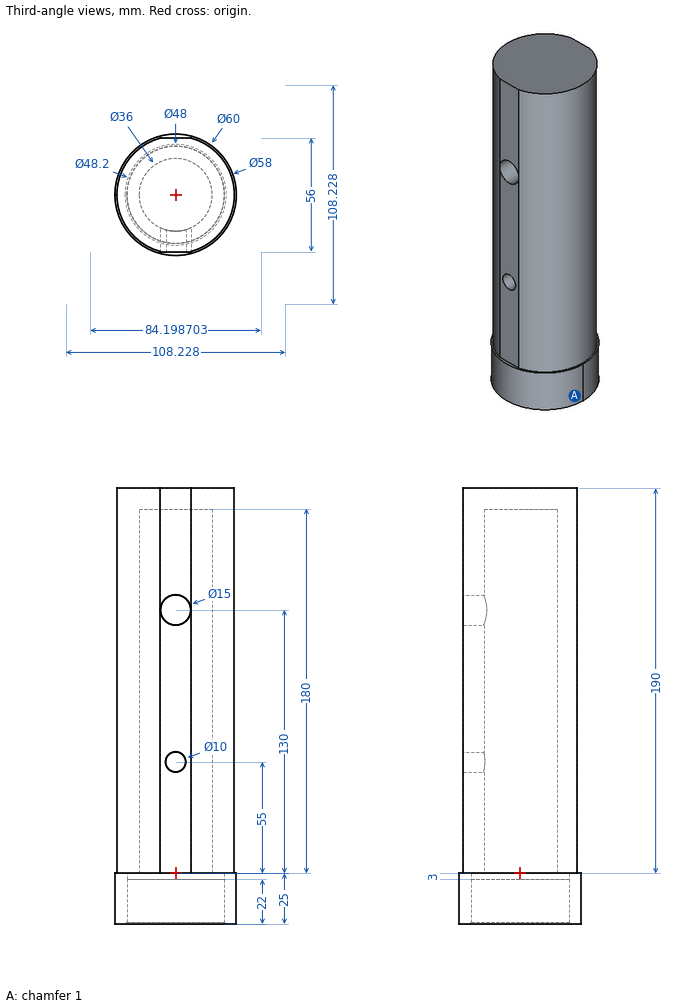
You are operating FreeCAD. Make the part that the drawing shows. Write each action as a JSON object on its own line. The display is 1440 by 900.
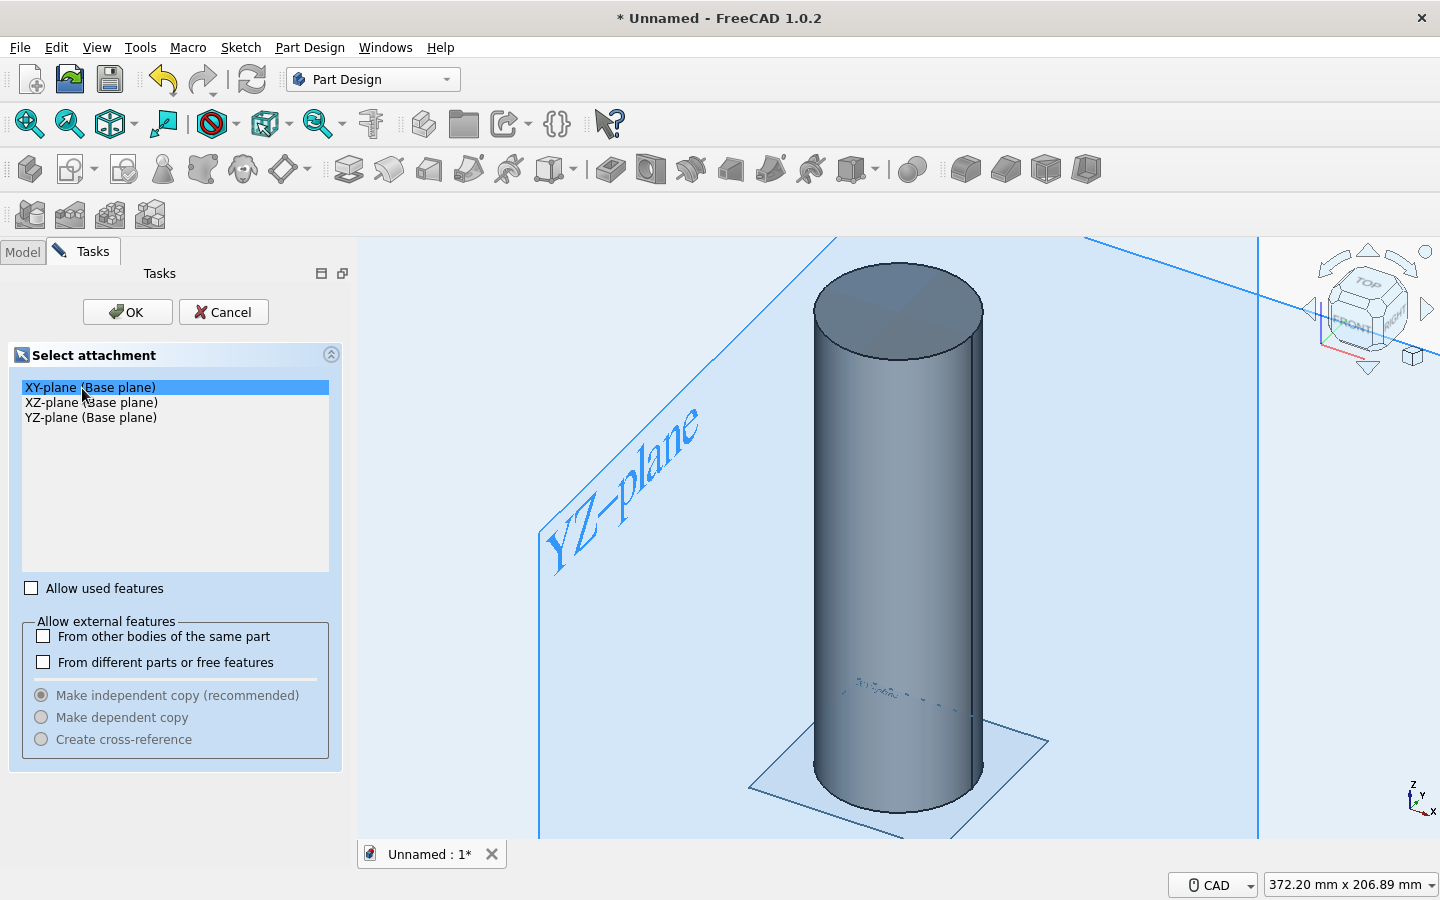
{"action": "left_click", "coordinate": [128, 312]}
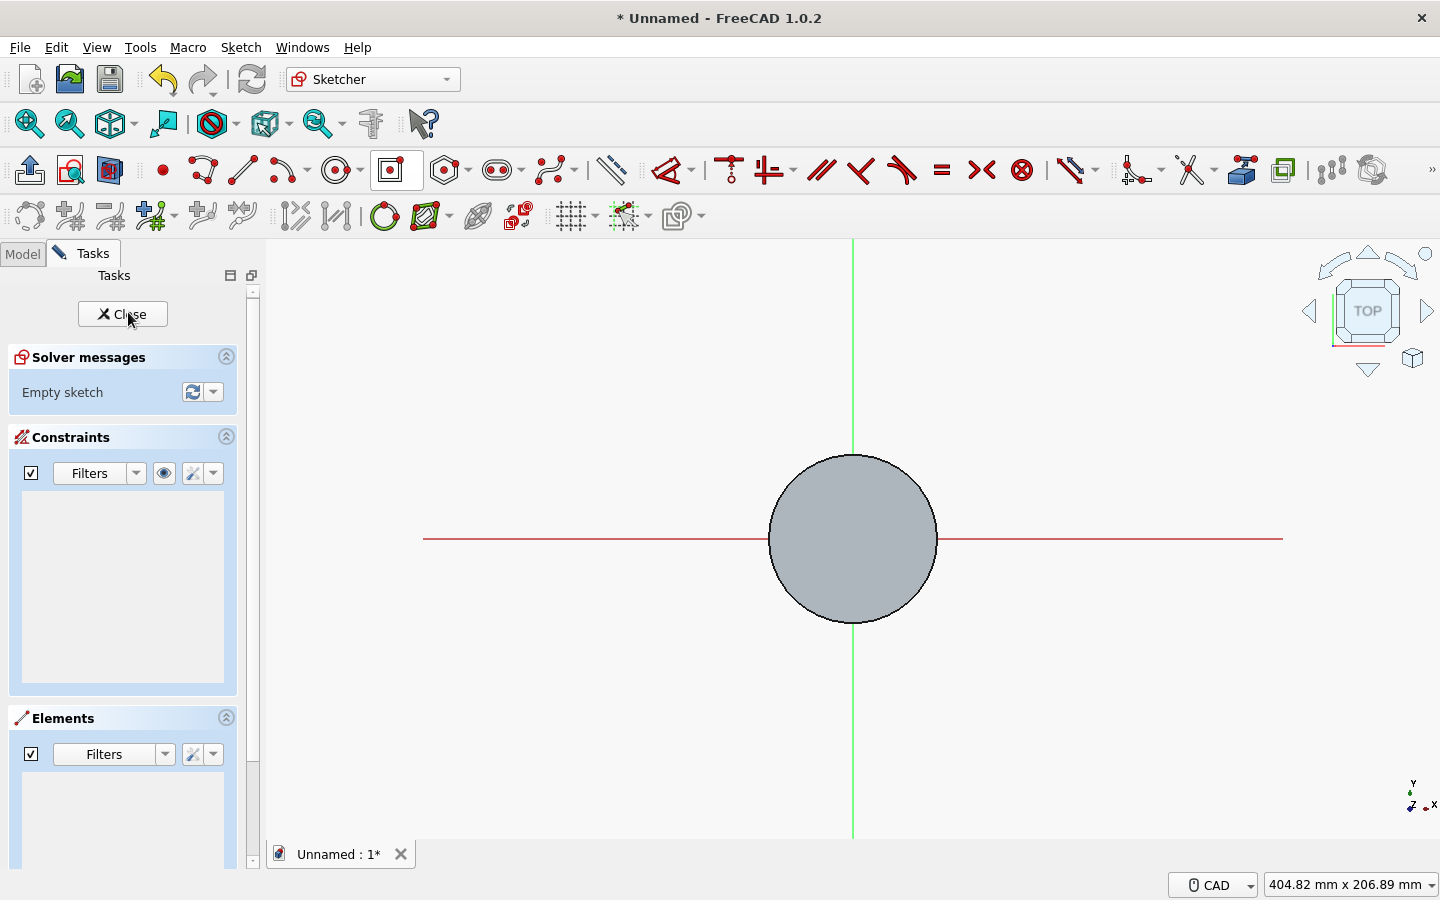
{"action": "left_click", "coordinate": [110, 170]}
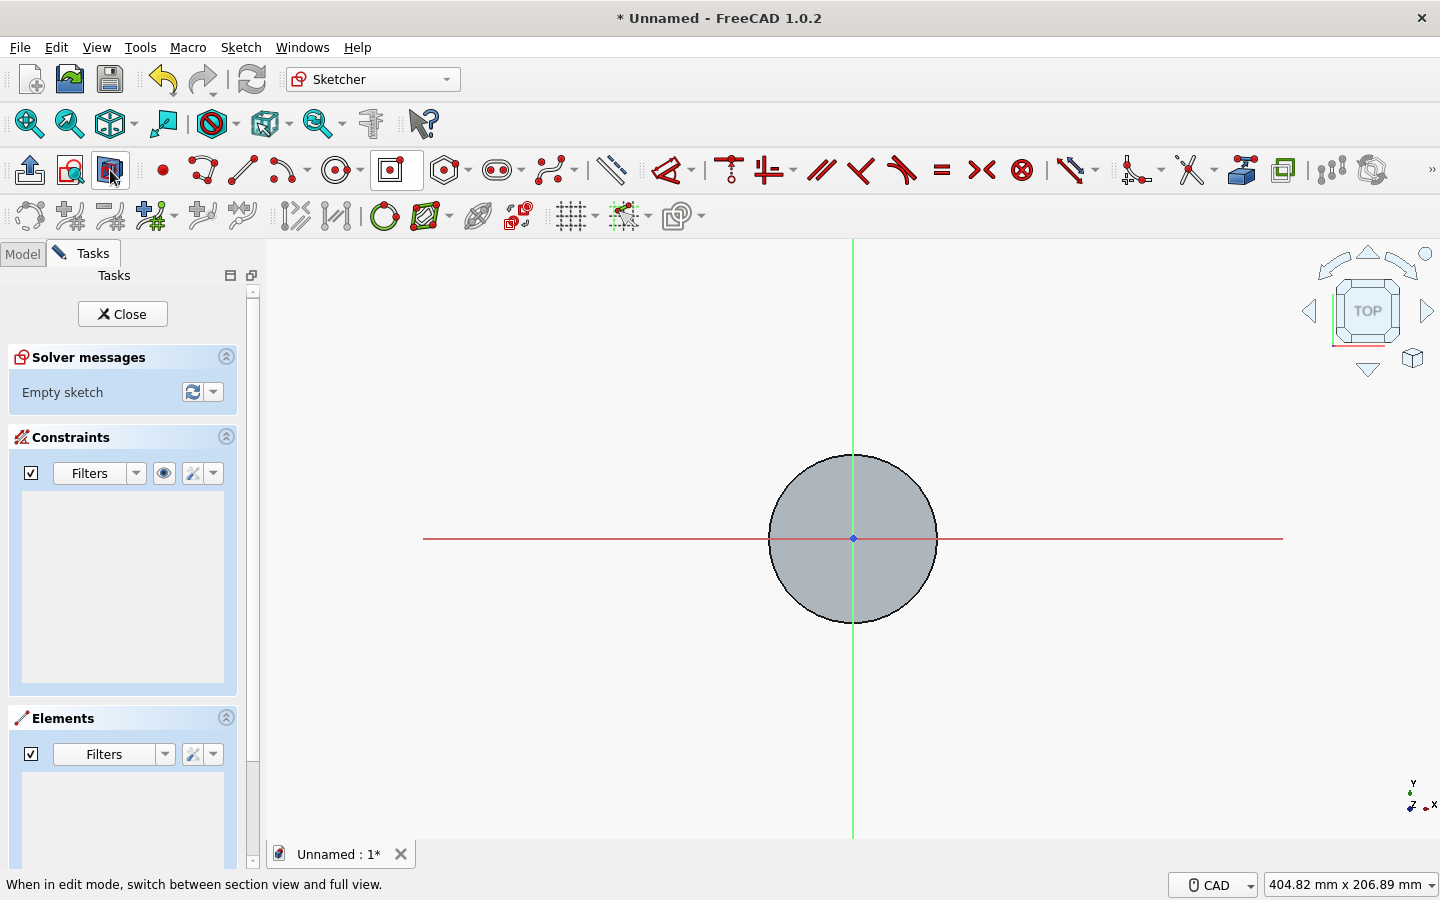
{"action": "scroll", "coordinate": [909, 539], "scroll_direction": "up", "scroll_amount": 4}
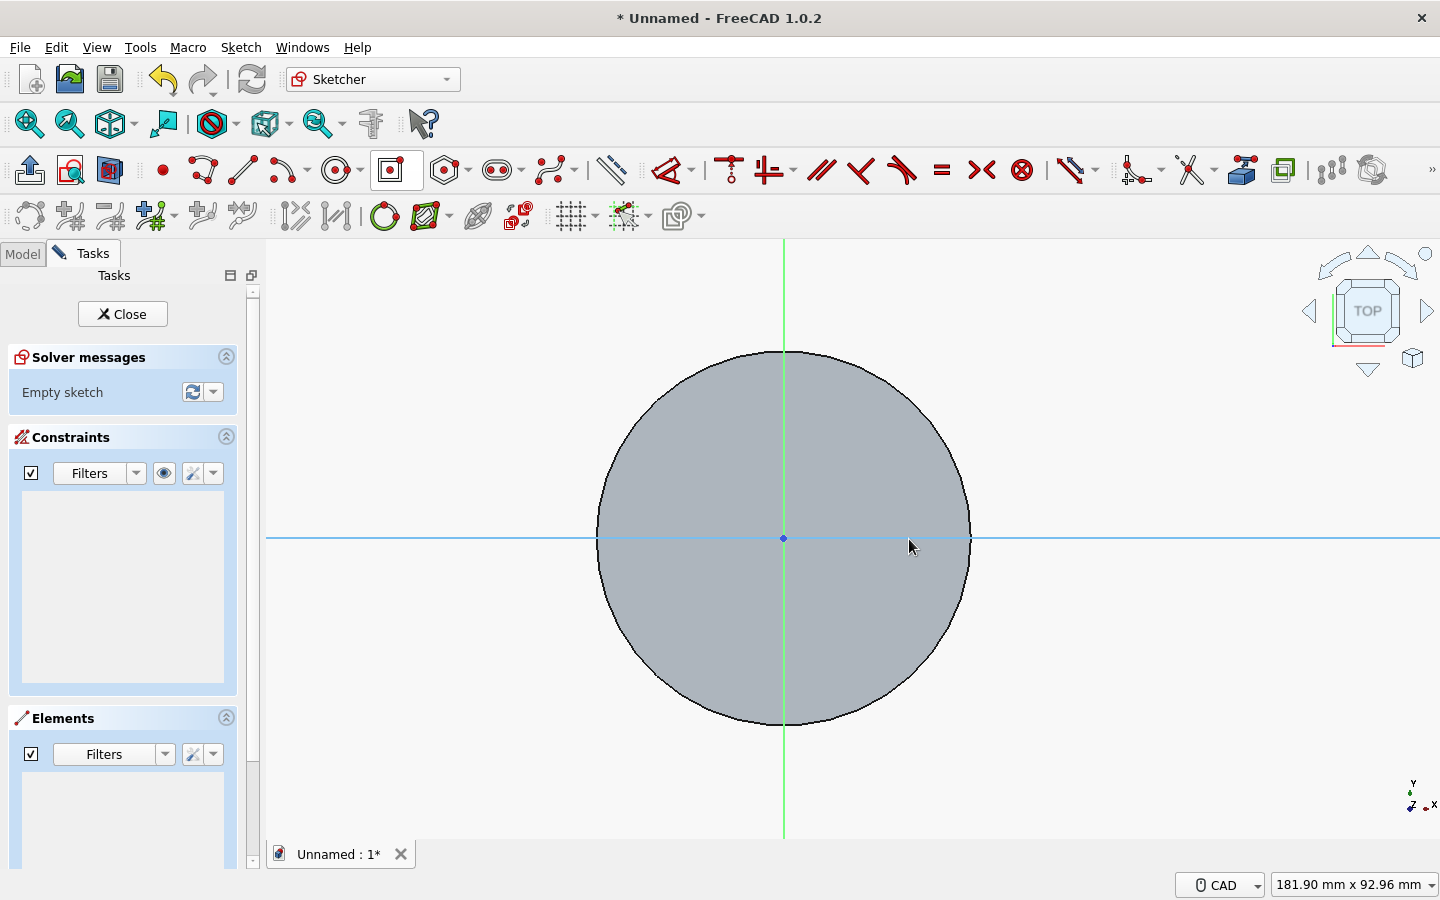
{"action": "left_click", "coordinate": [336, 170]}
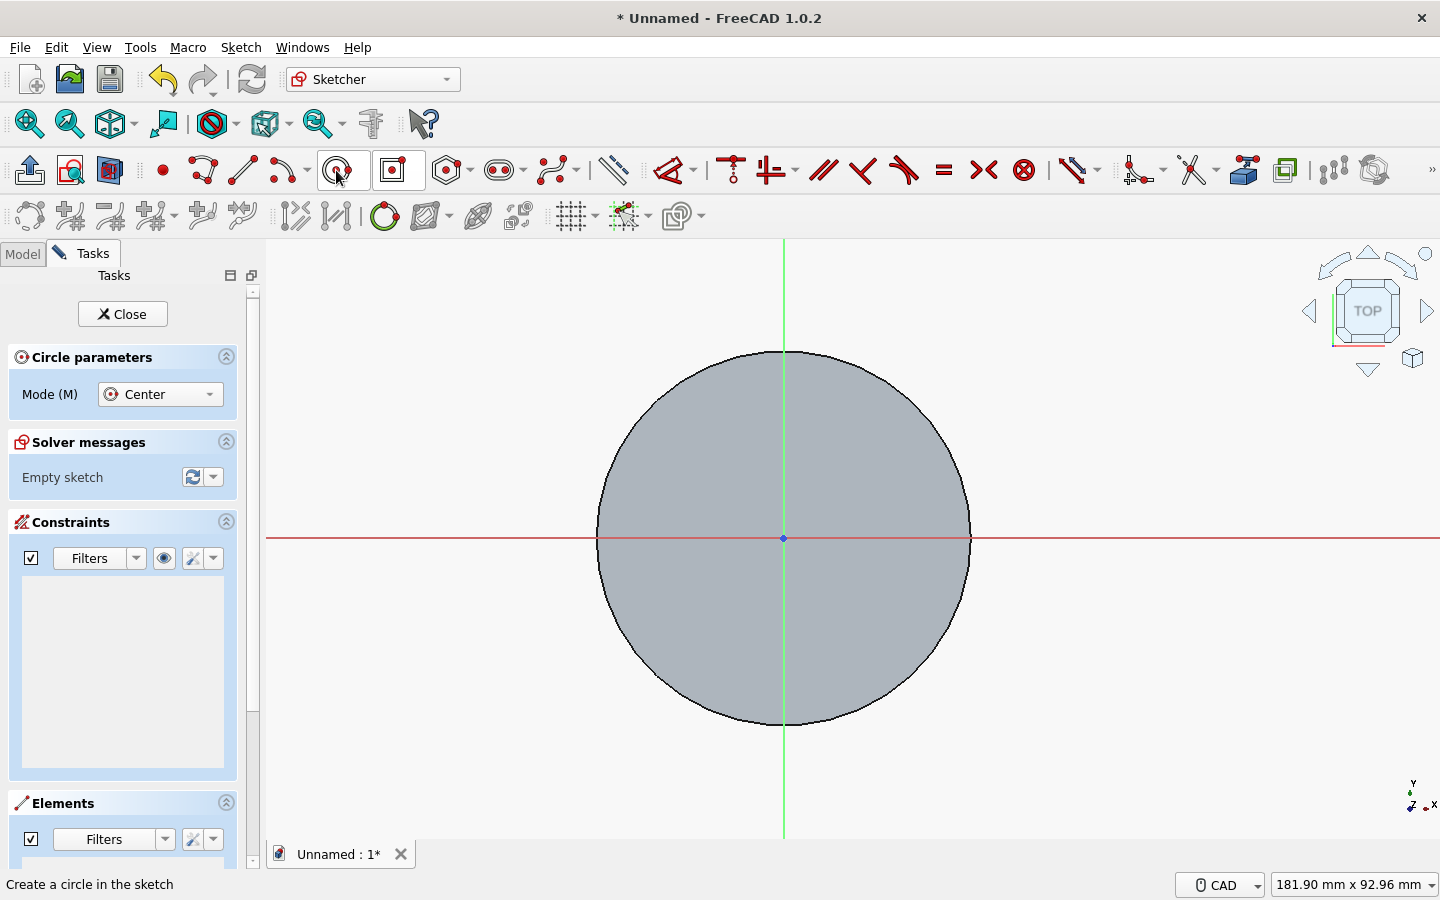
{"action": "left_click", "coordinate": [784, 538]}
{"action": "left_click", "coordinate": [921, 401]}
{"action": "key", "text": "Escape"}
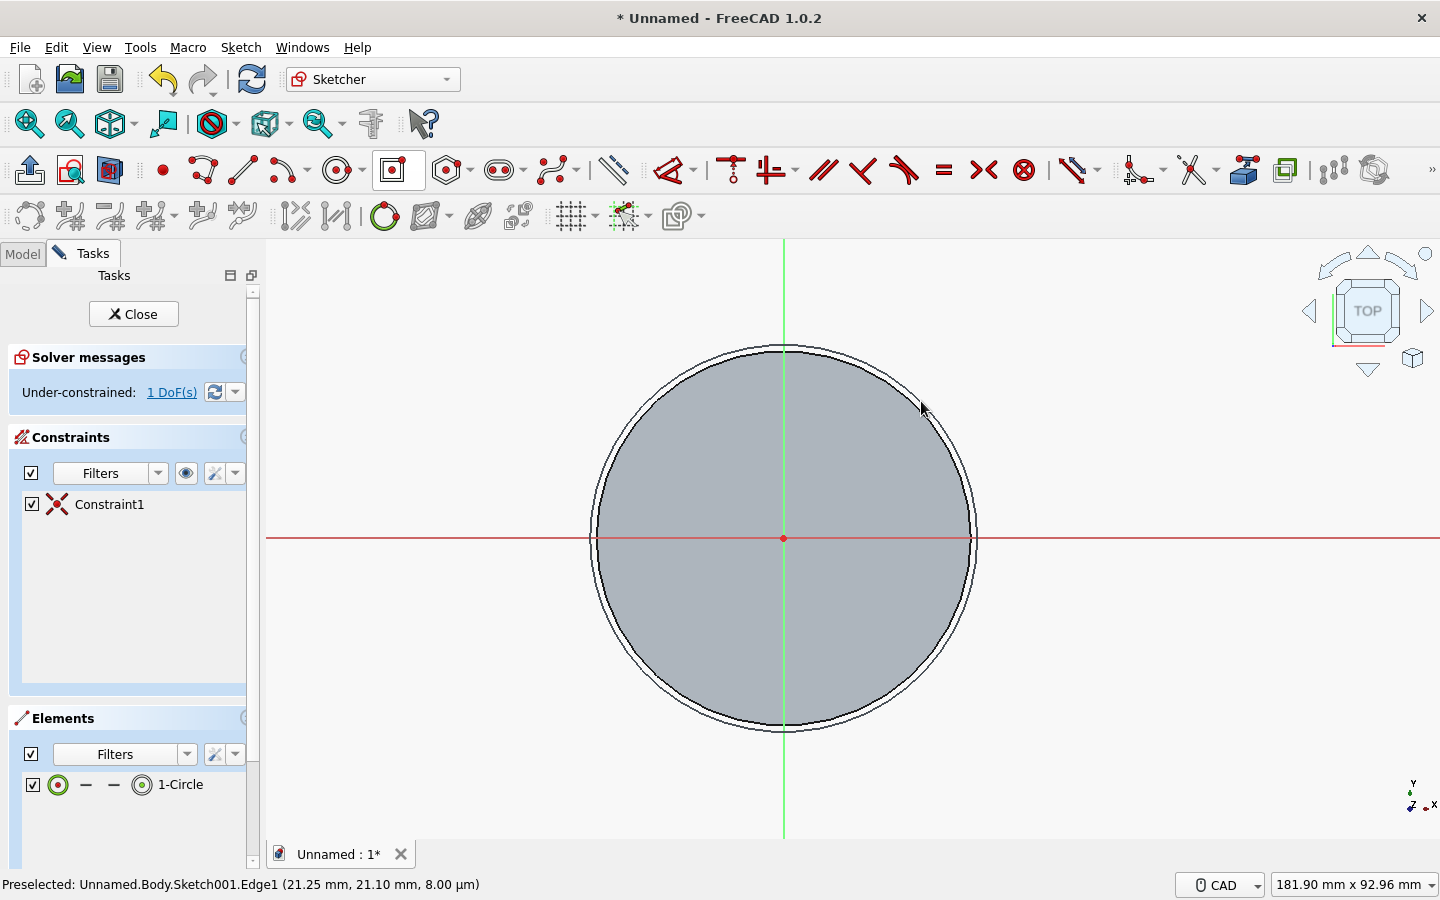
{"action": "left_click", "coordinate": [920, 401]}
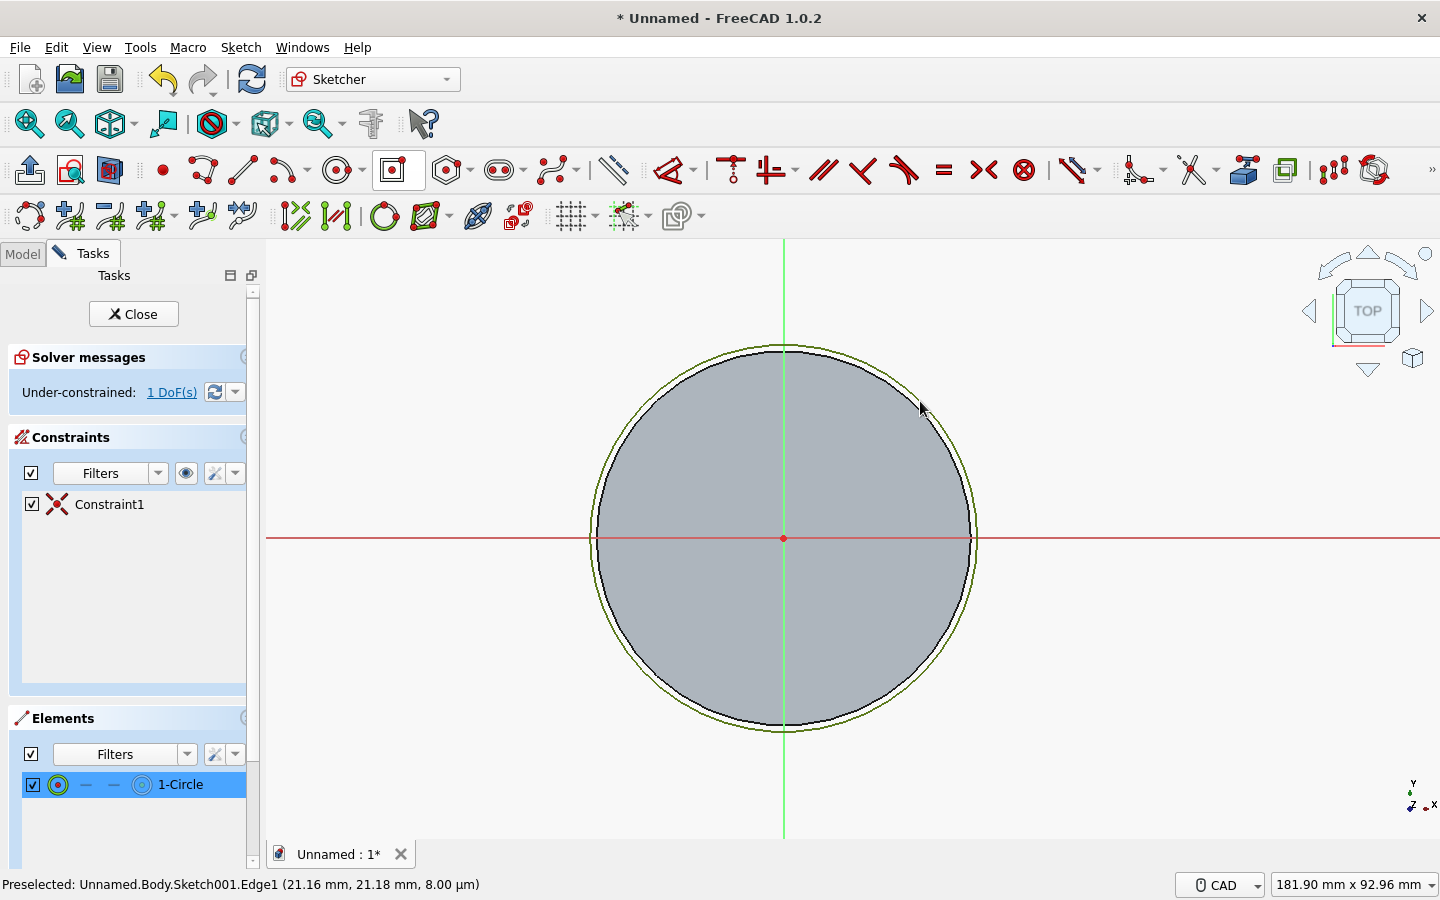
{"action": "left_click", "coordinate": [696, 170]}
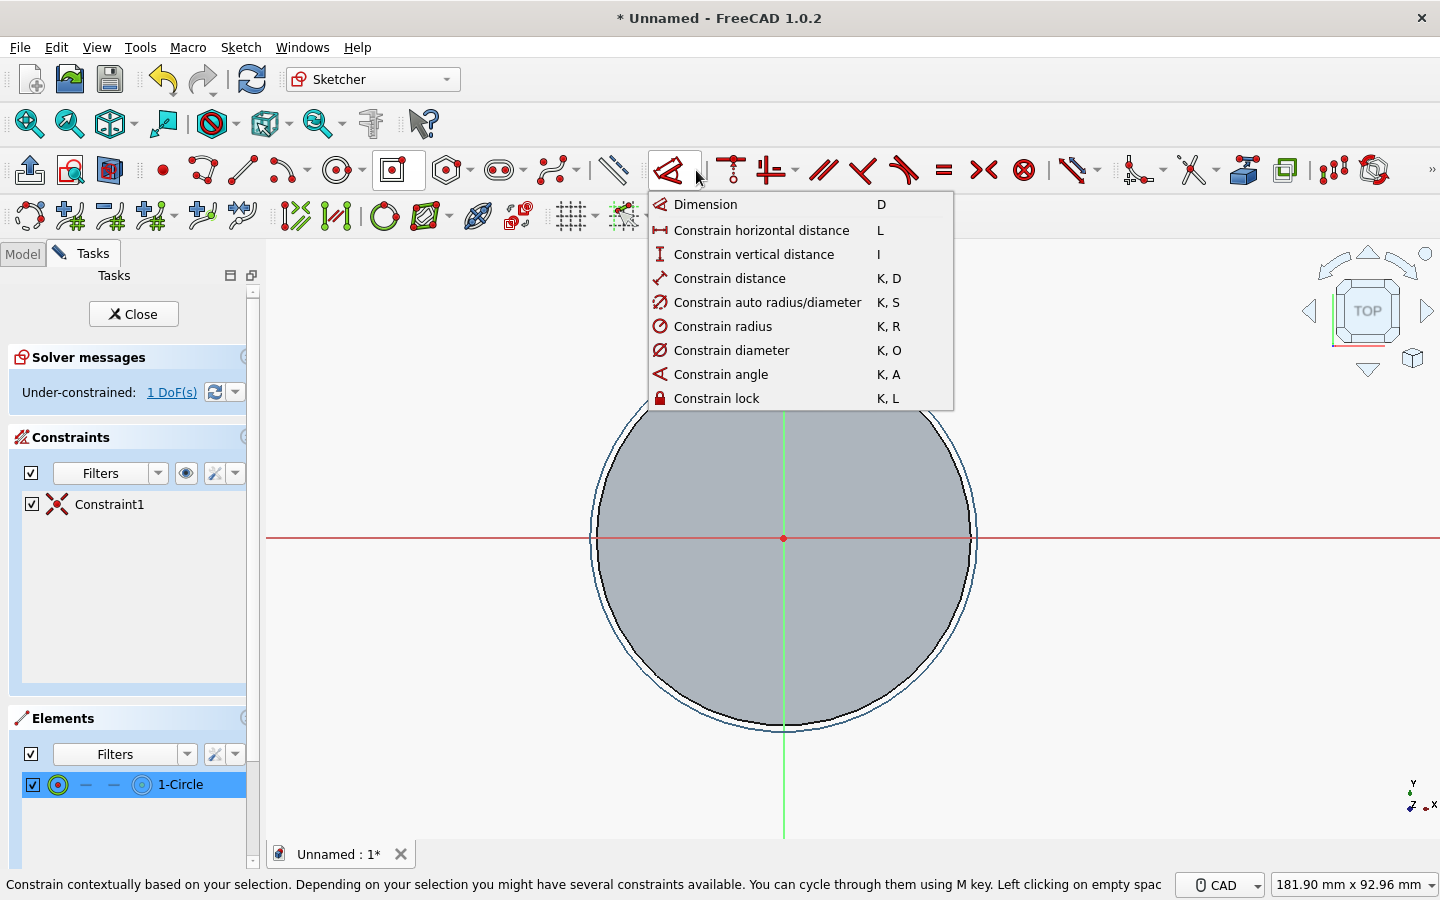
{"action": "left_click", "coordinate": [801, 350]}